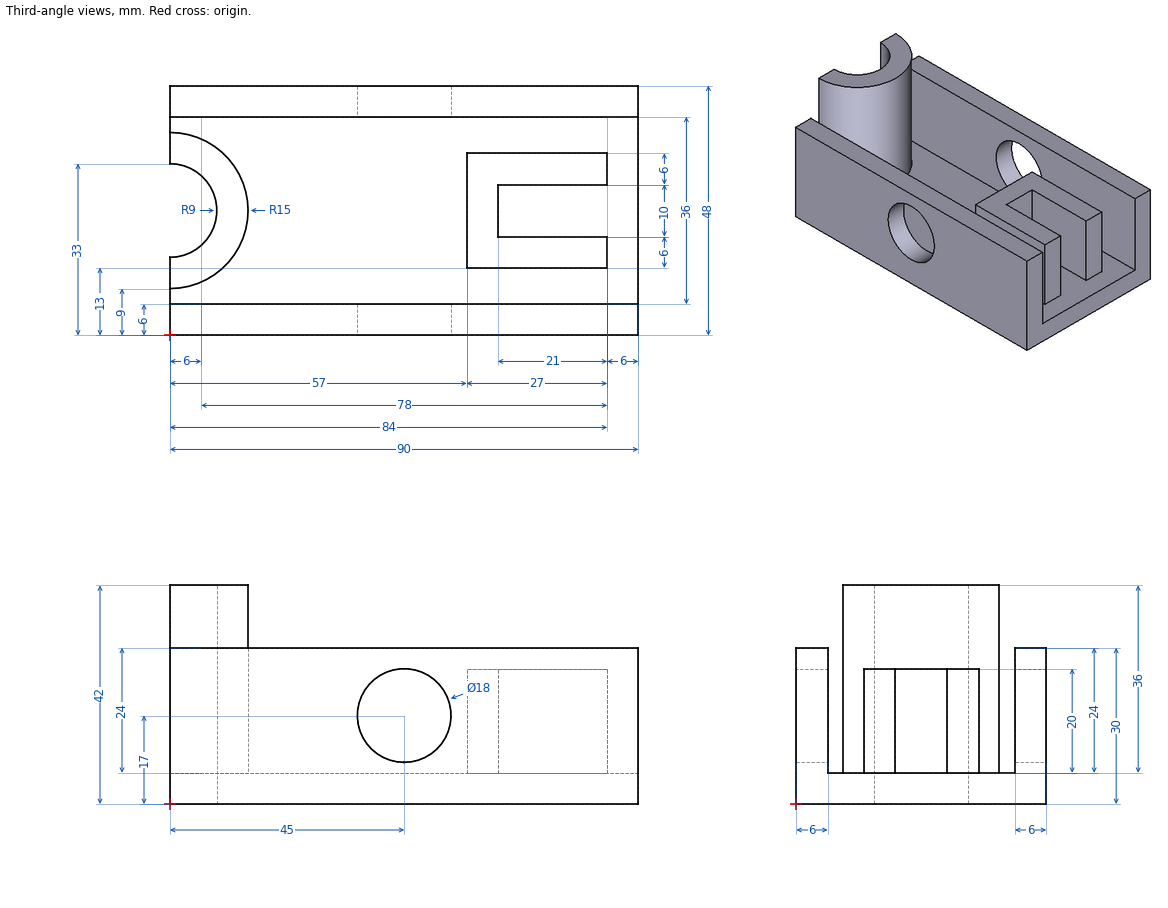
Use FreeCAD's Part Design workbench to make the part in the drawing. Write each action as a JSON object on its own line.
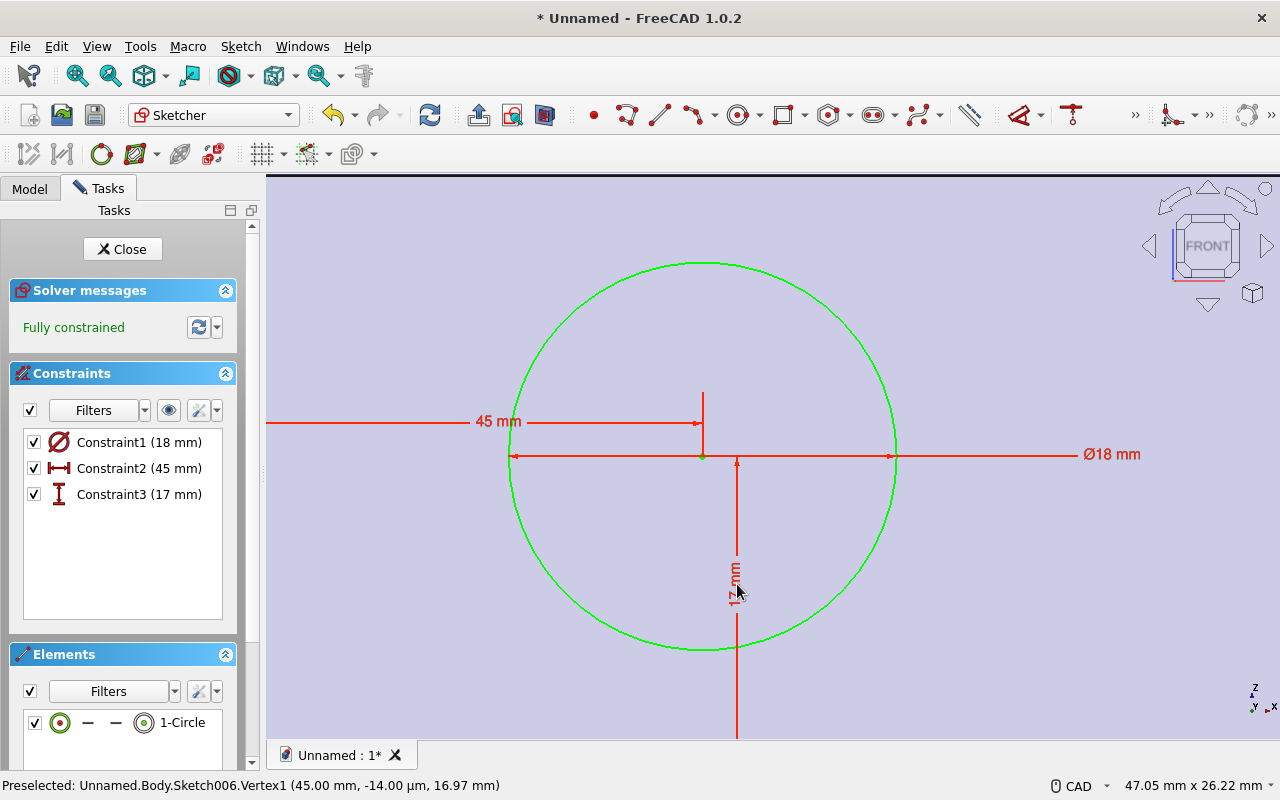
{"action": "left_click", "coordinate": [123, 249]}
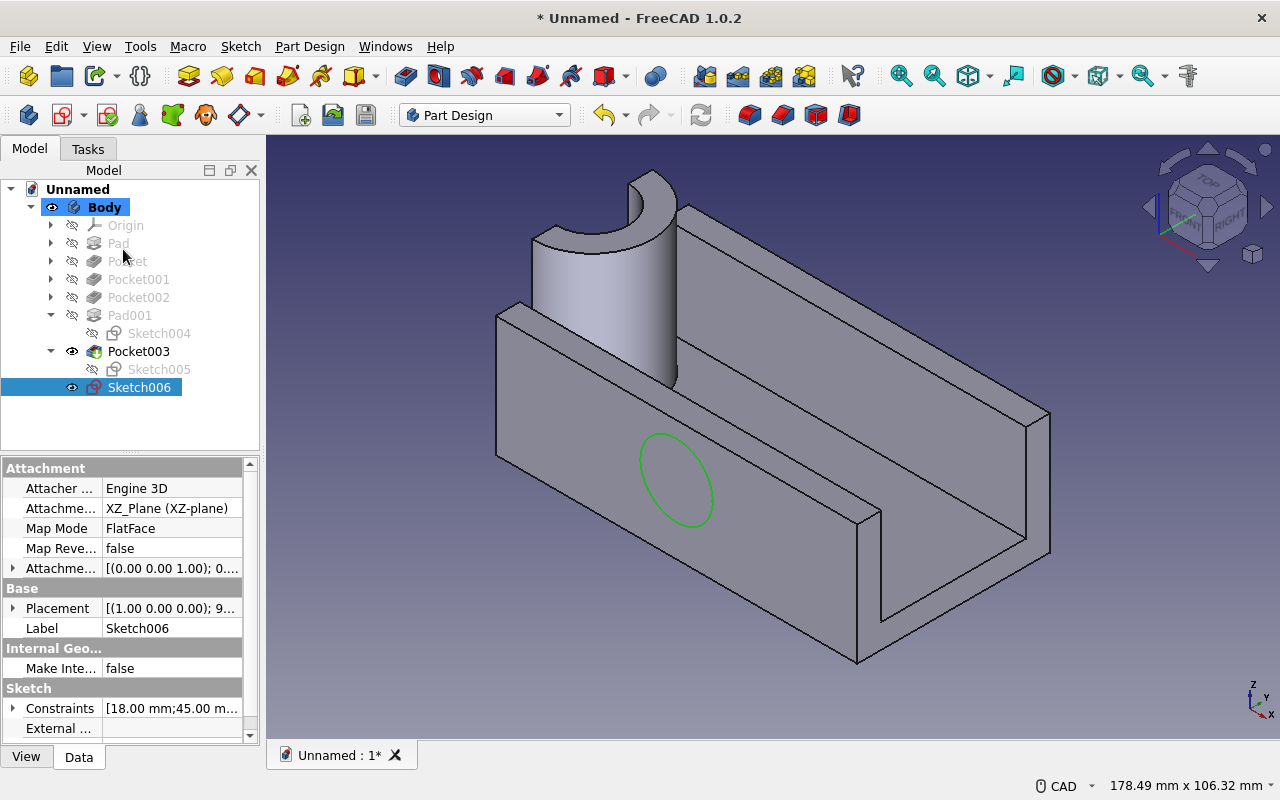
{"action": "left_click", "coordinate": [406, 76]}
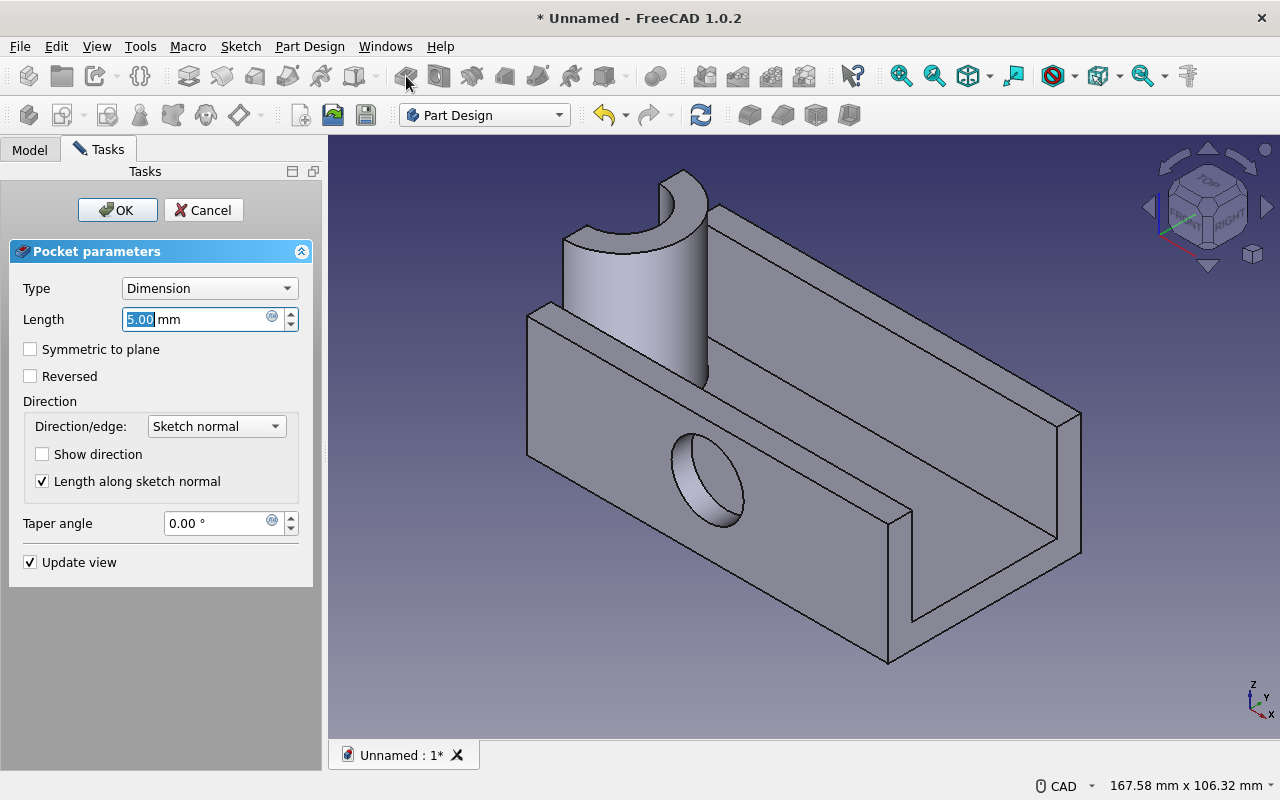
{"action": "type", "text": "6"}
{"action": "key", "text": "Tab"}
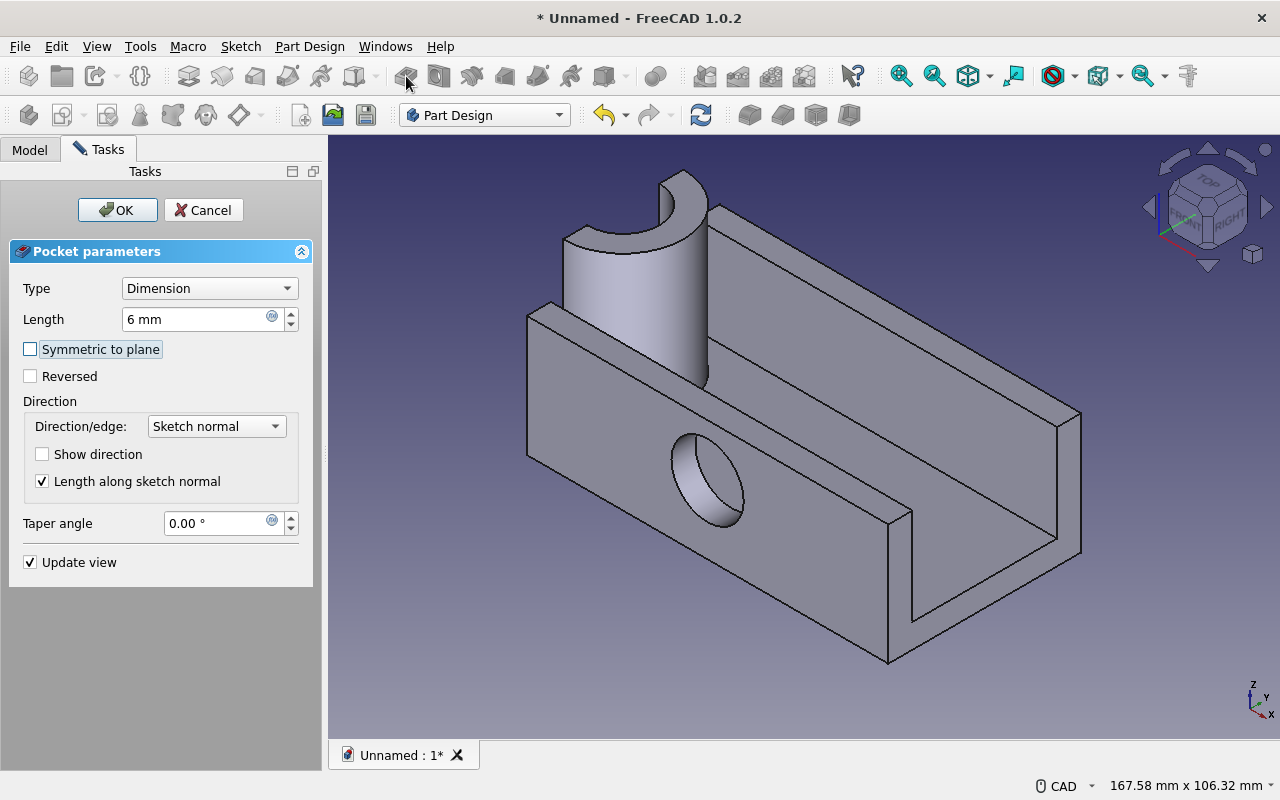
{"action": "left_click", "coordinate": [118, 210]}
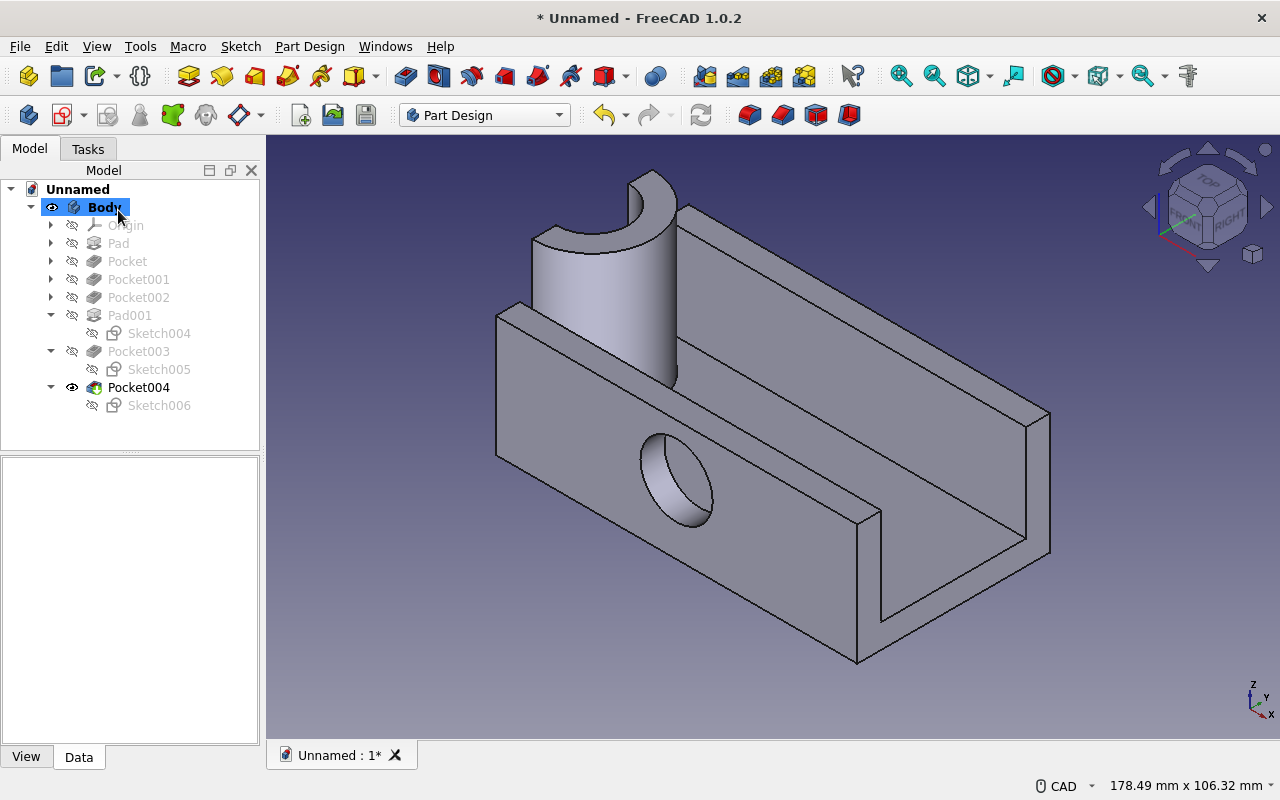
{"action": "left_click", "coordinate": [845, 377]}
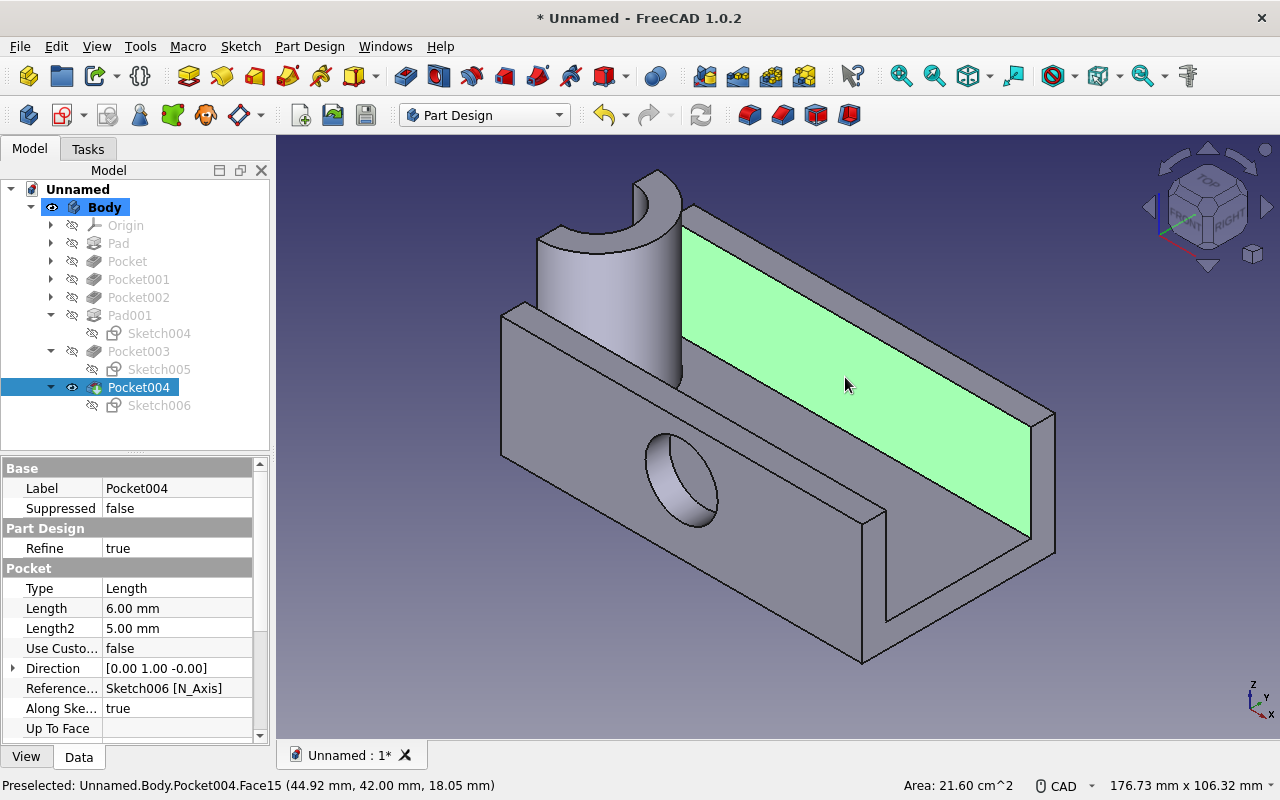
{"action": "left_click", "coordinate": [62, 116]}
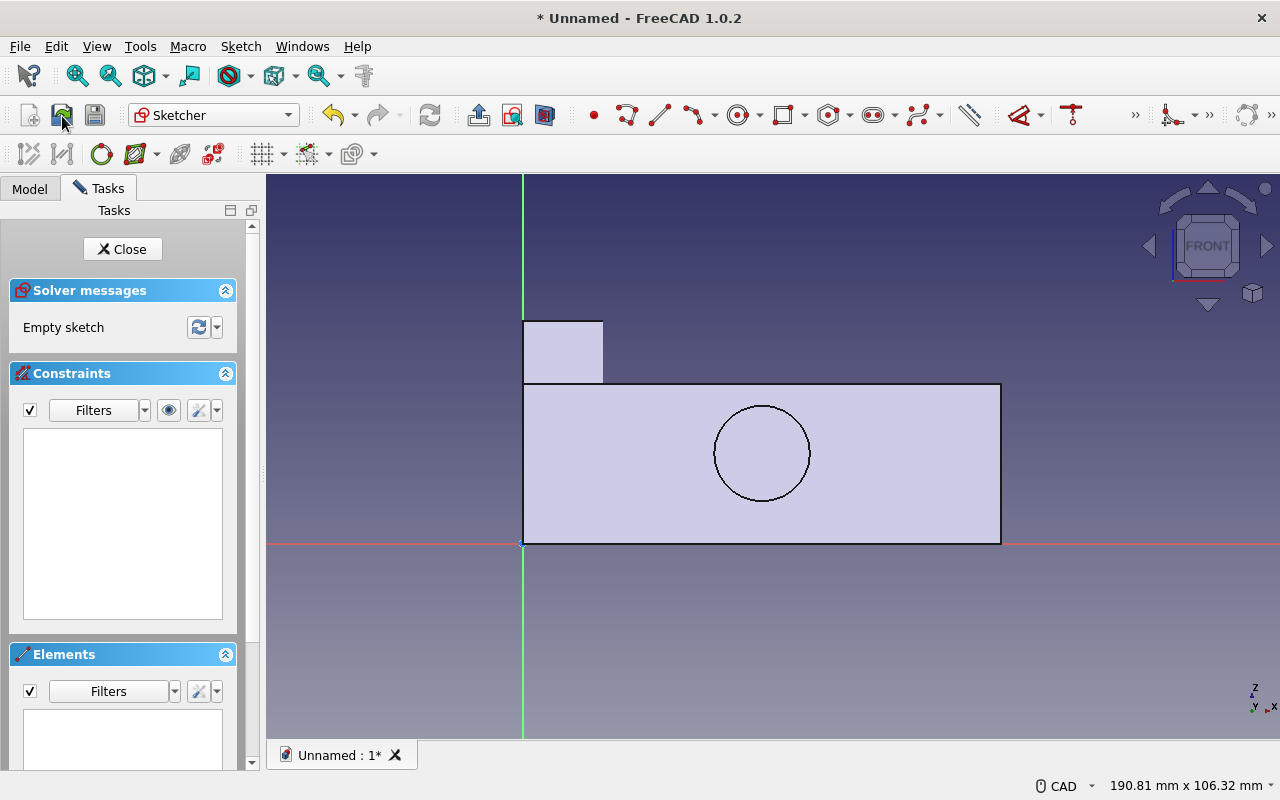
{"action": "scroll", "coordinate": [781, 452], "scroll_direction": "up", "scroll_amount": 7}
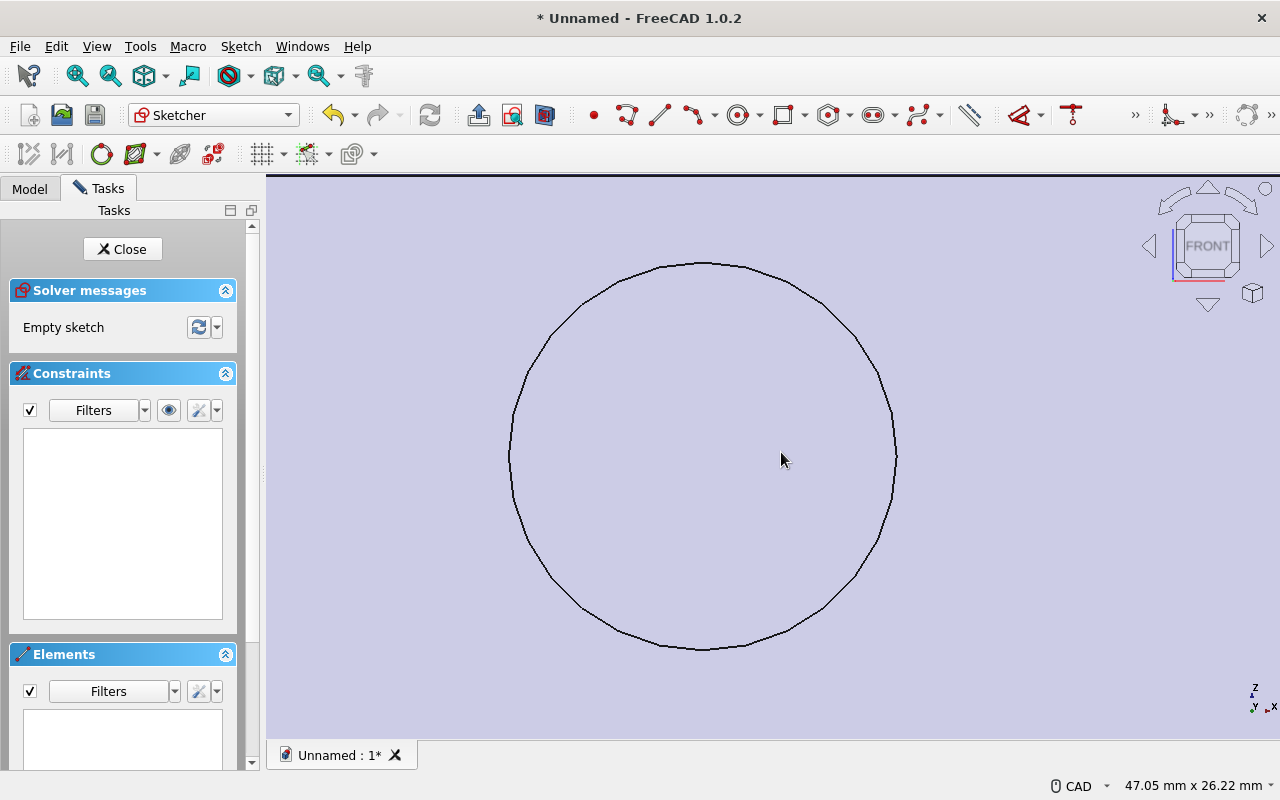
{"action": "key", "text": "g c"}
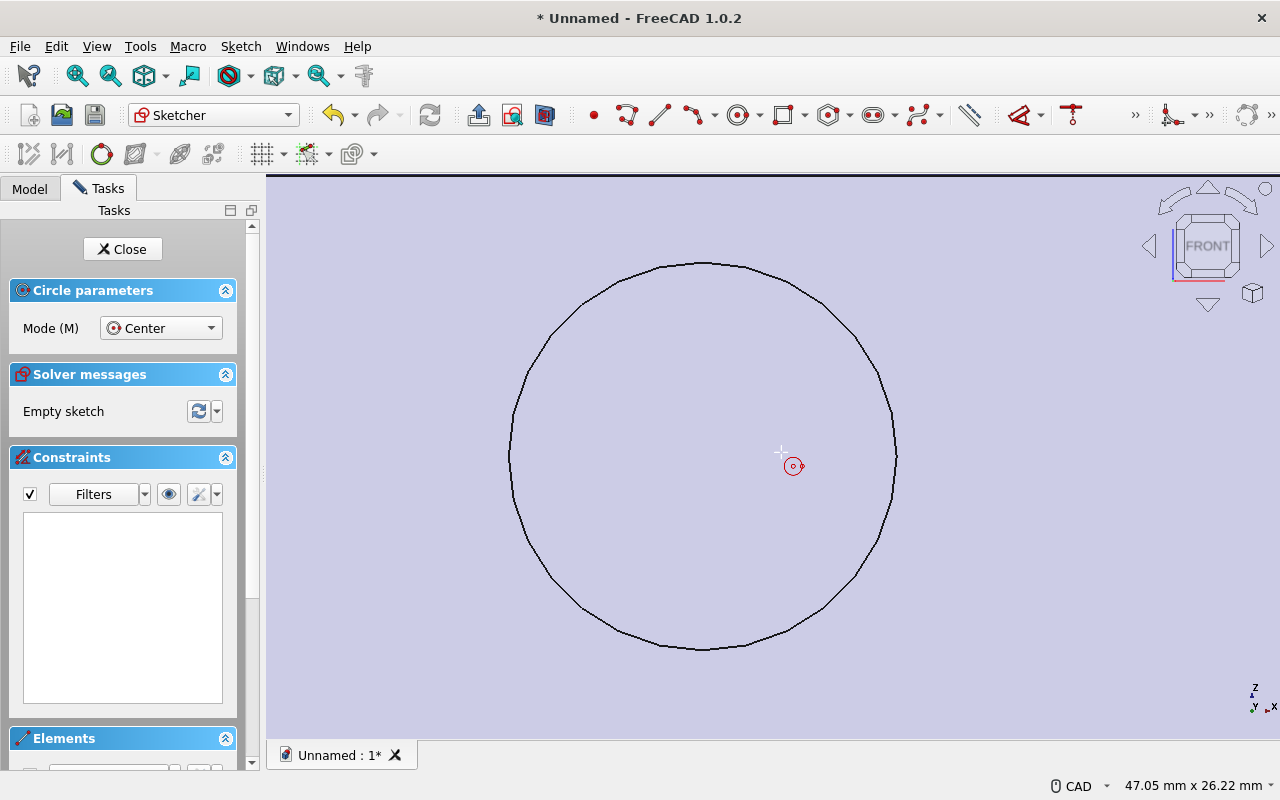
{"action": "left_click", "coordinate": [703, 456]}
{"action": "mouse_move", "coordinate": [840, 319]}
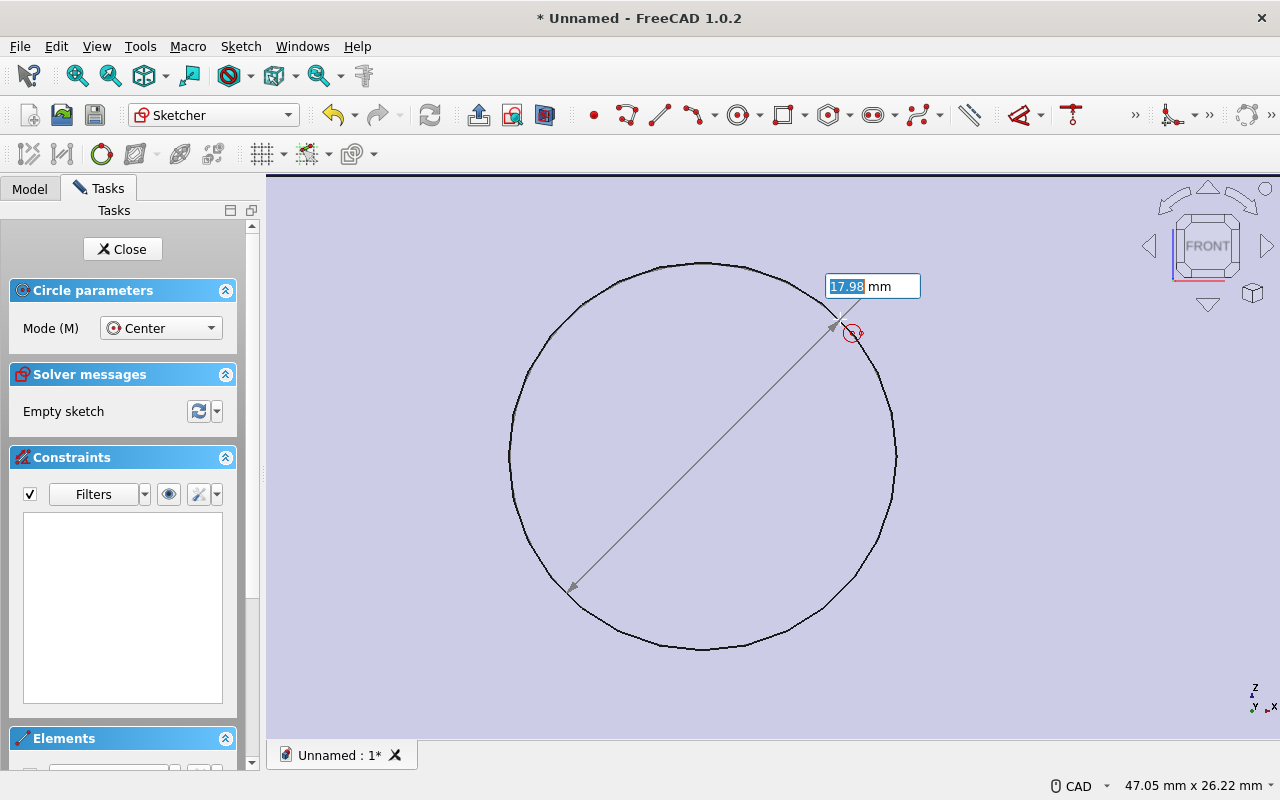
{"action": "type", "text": "18"}
{"action": "key", "text": "Return"}
{"action": "key", "text": "Escape"}